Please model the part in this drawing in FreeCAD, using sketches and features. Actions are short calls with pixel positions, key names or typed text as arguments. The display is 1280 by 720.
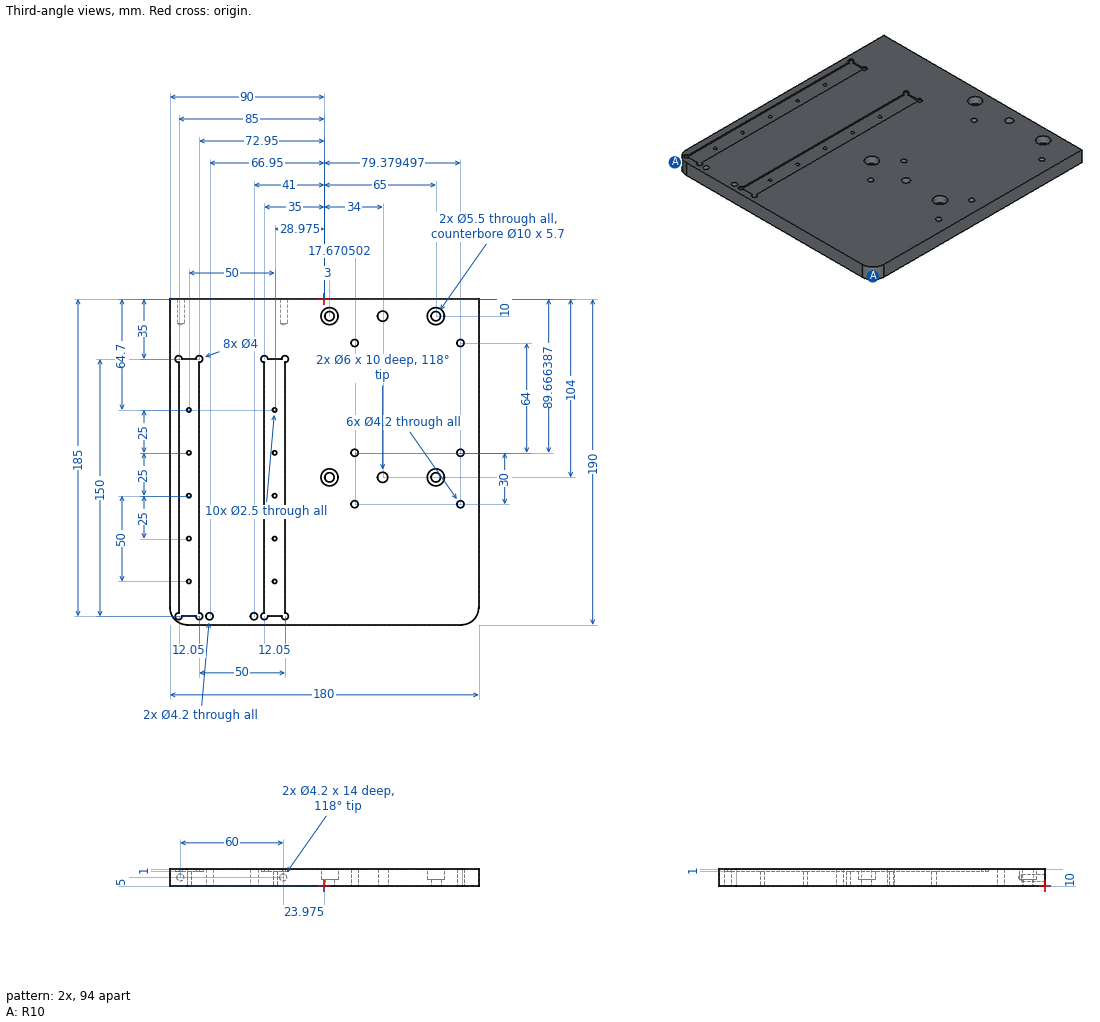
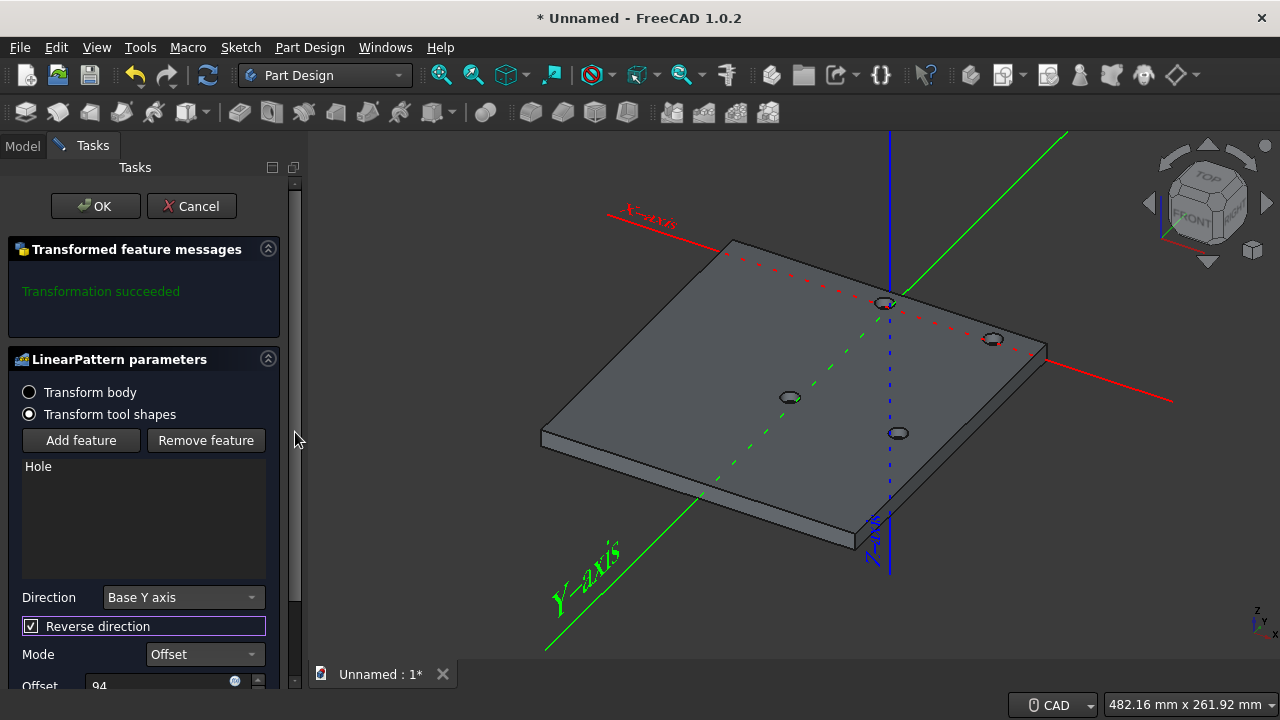
click(96, 206)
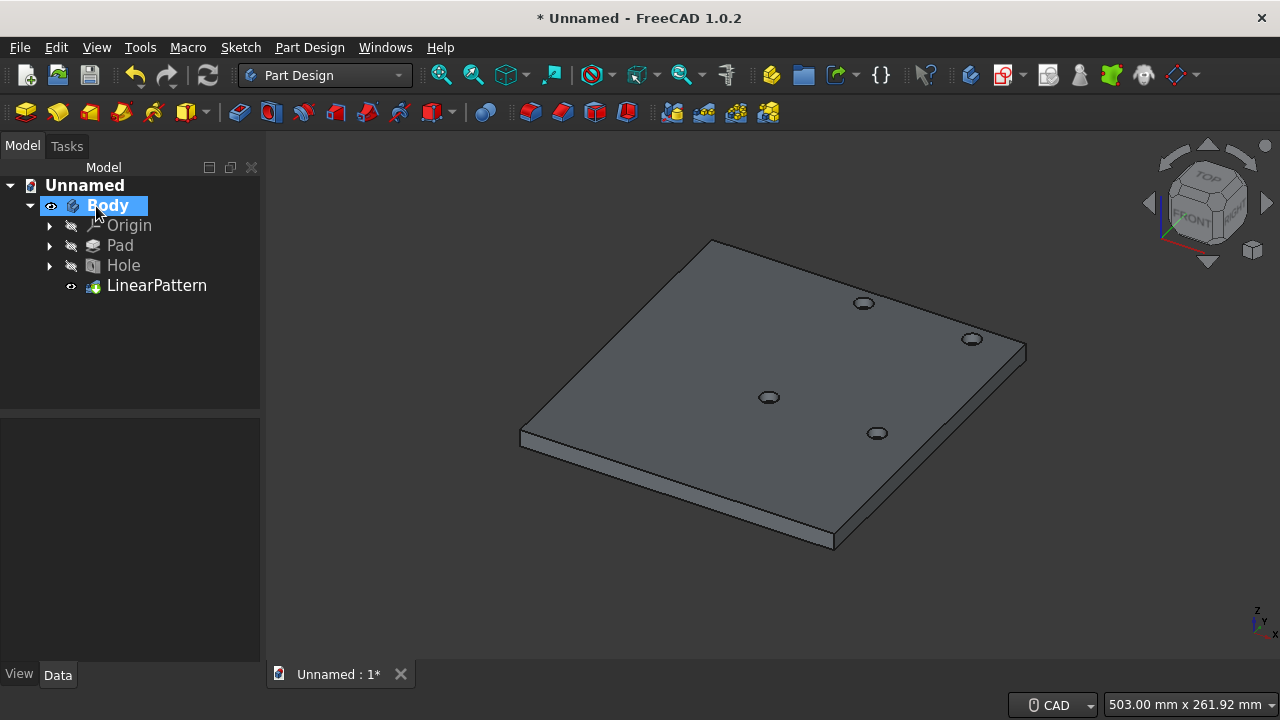
click(755, 344)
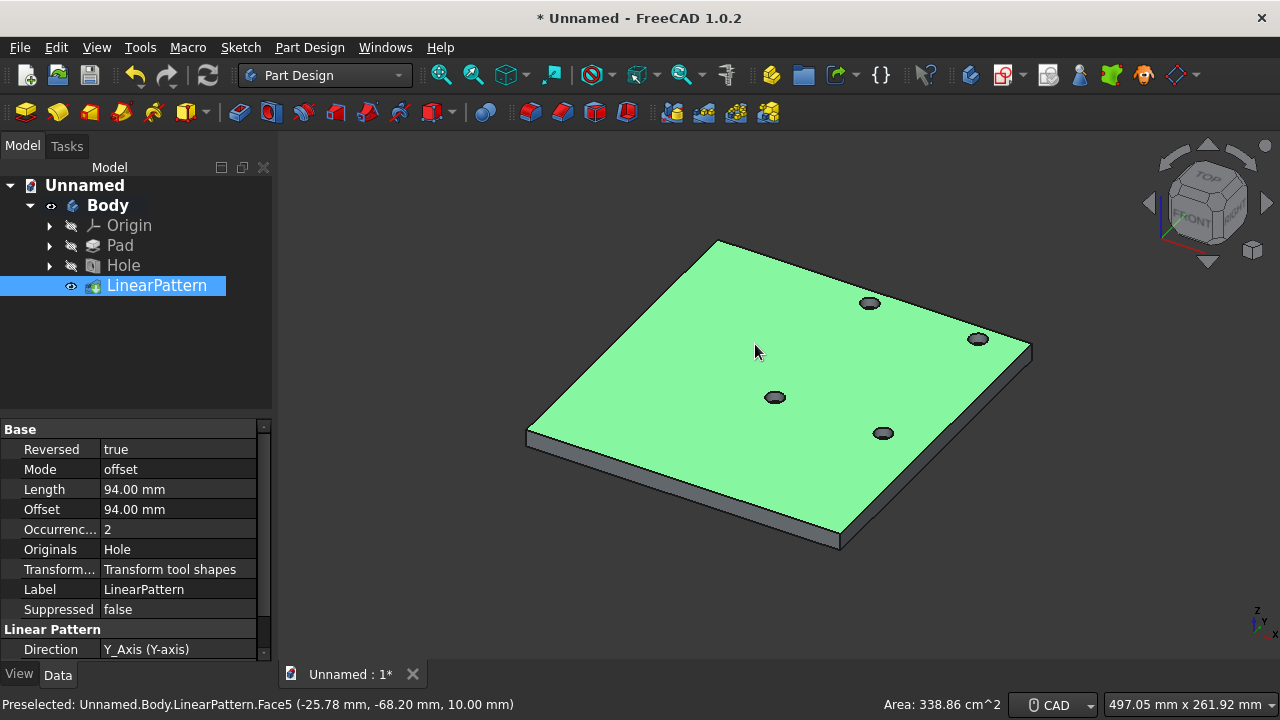
click(1004, 76)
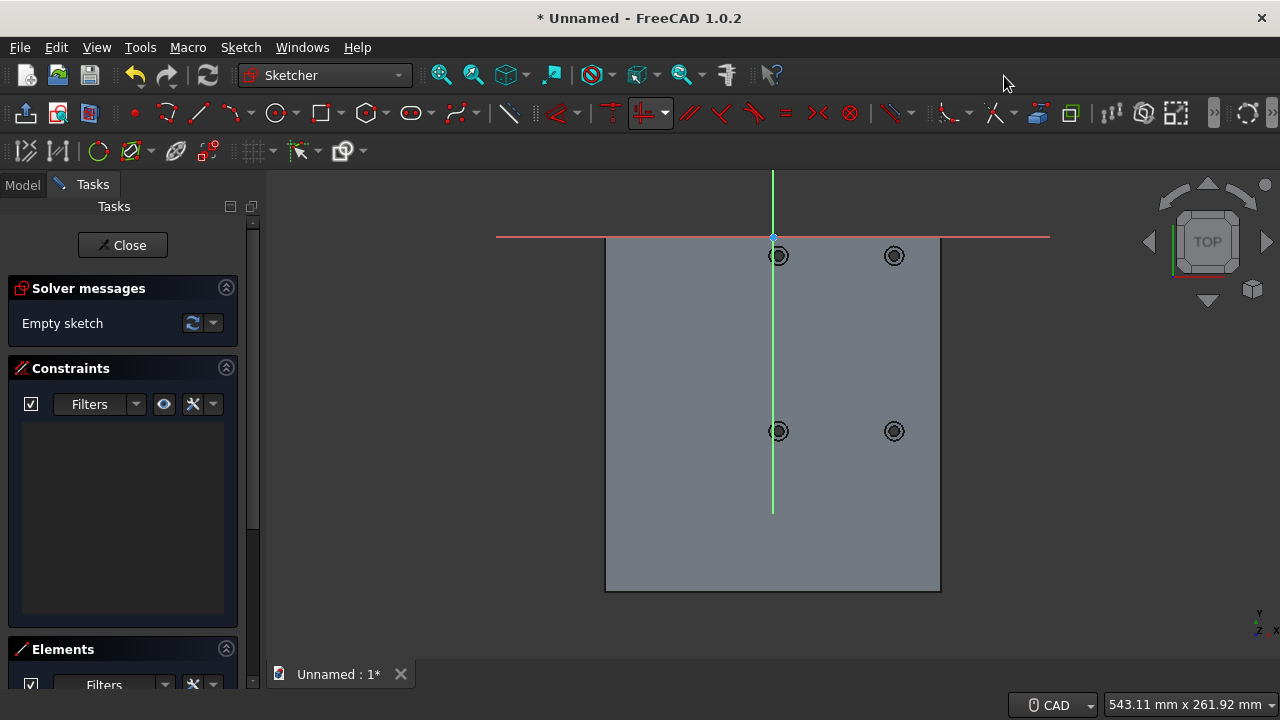
click(322, 114)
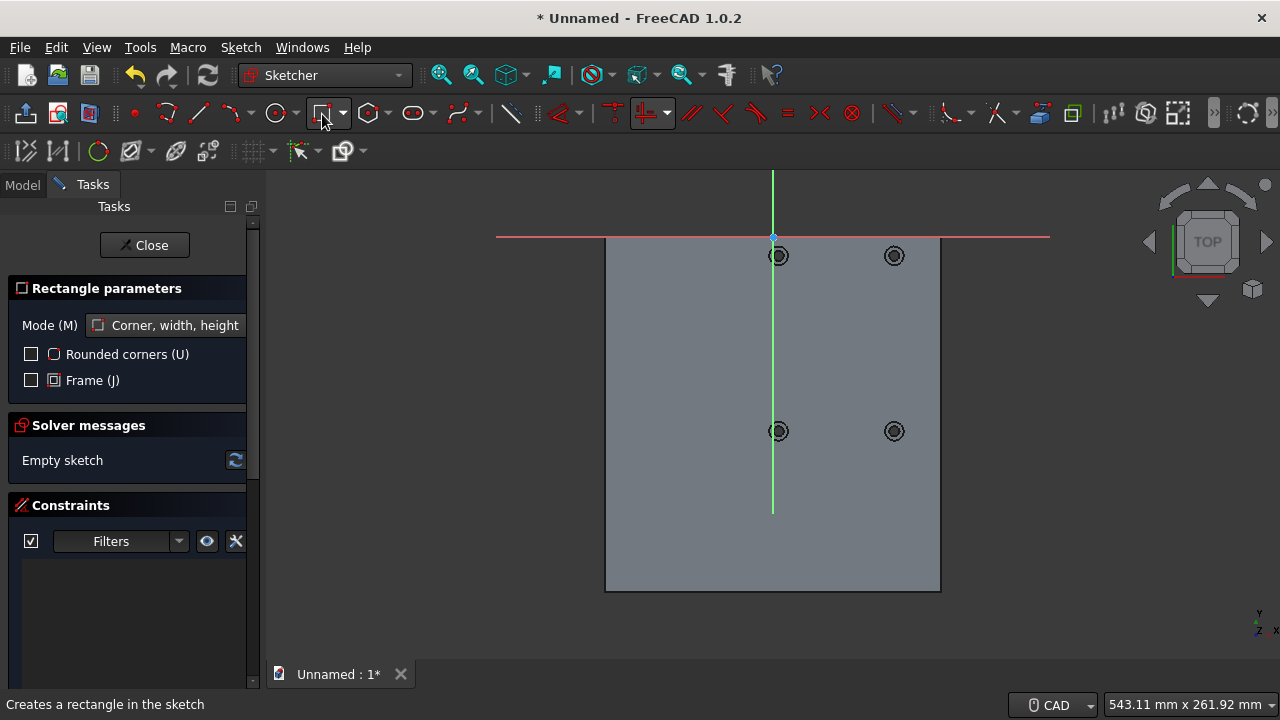
click(614, 302)
move(637, 583)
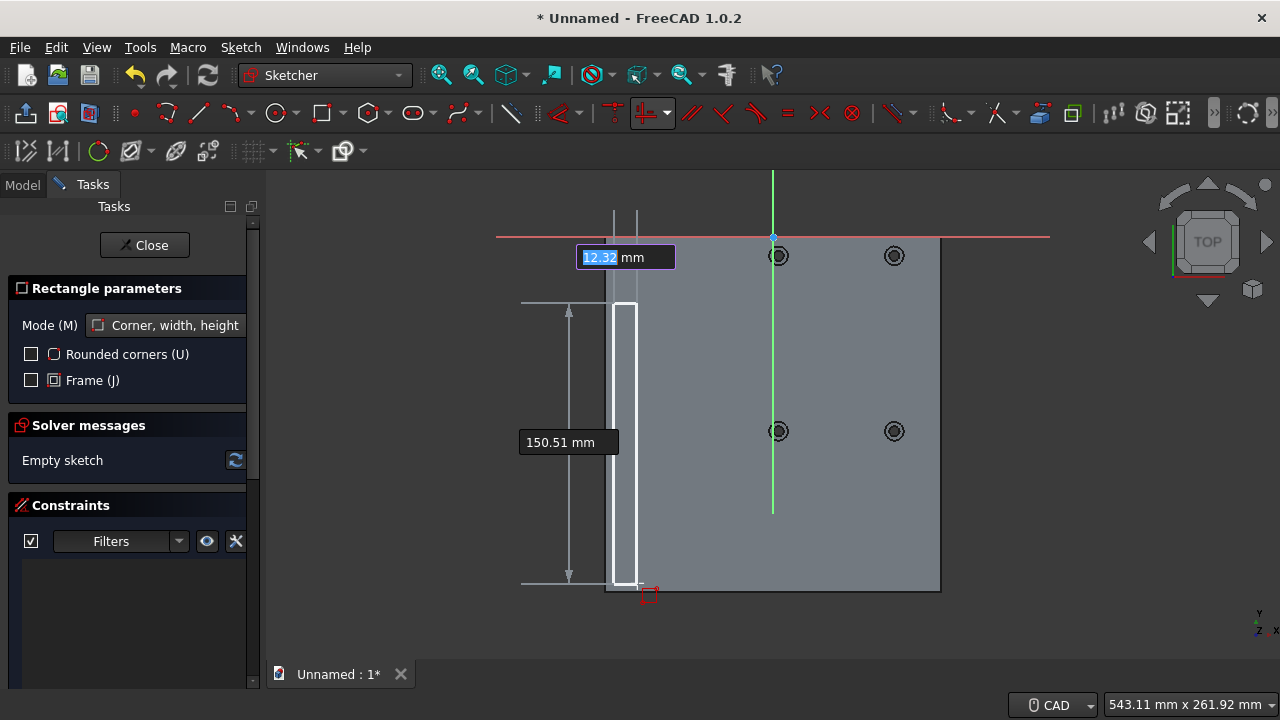
text(12.05)
key(Tab)
text(150)
key(Return)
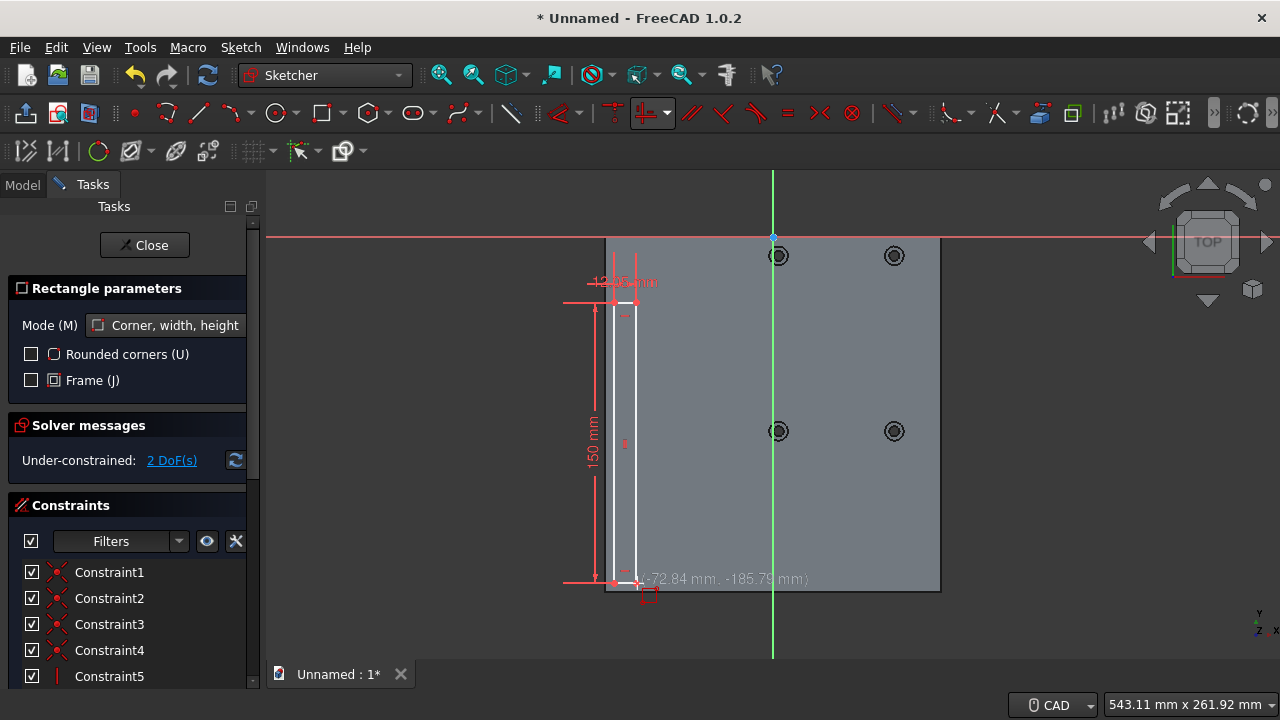
click(708, 302)
move(730, 583)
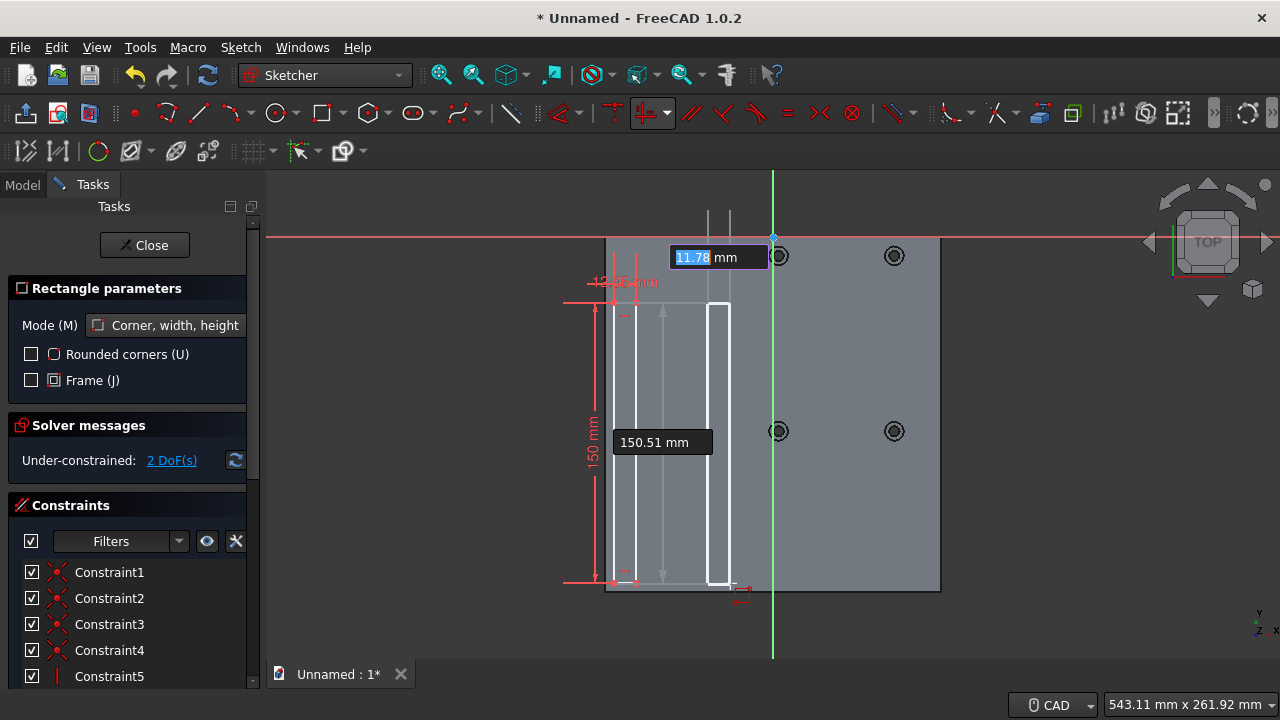
text(12.05)
key(Tab)
text(150)
key(Return)
key(Escape)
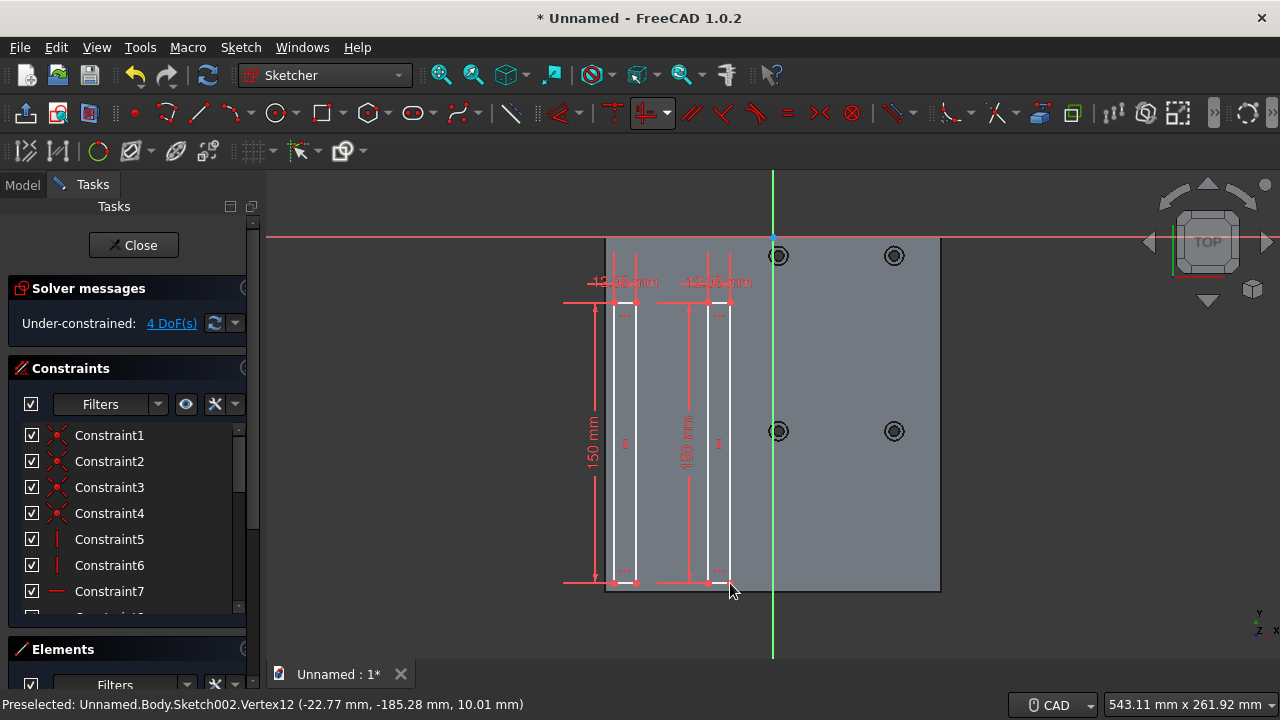
click(614, 303)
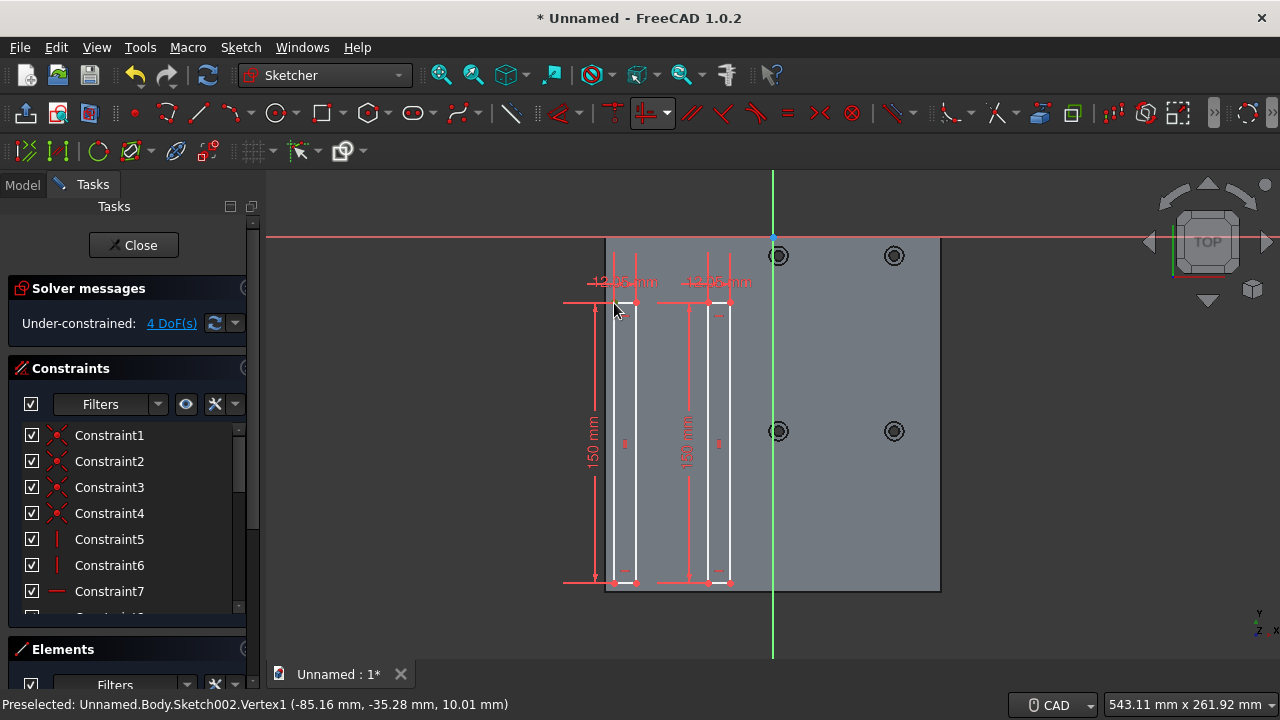
key(l)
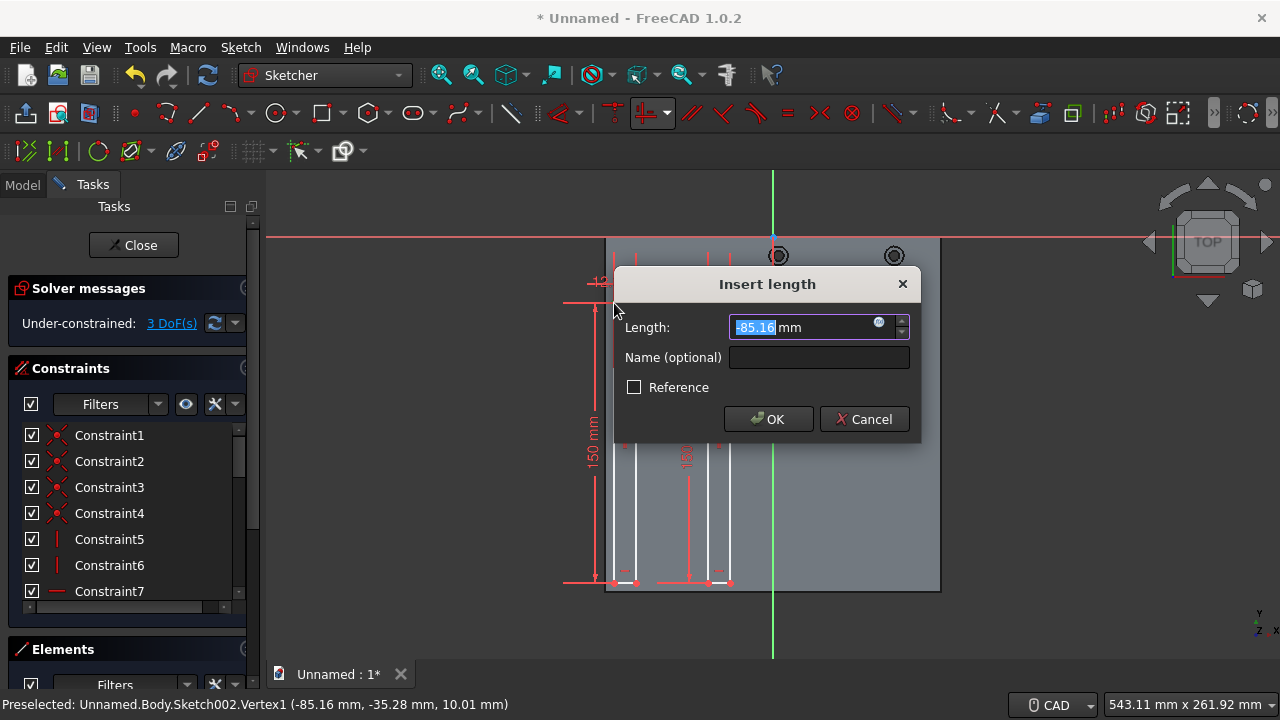
text(-85)
key(Return)